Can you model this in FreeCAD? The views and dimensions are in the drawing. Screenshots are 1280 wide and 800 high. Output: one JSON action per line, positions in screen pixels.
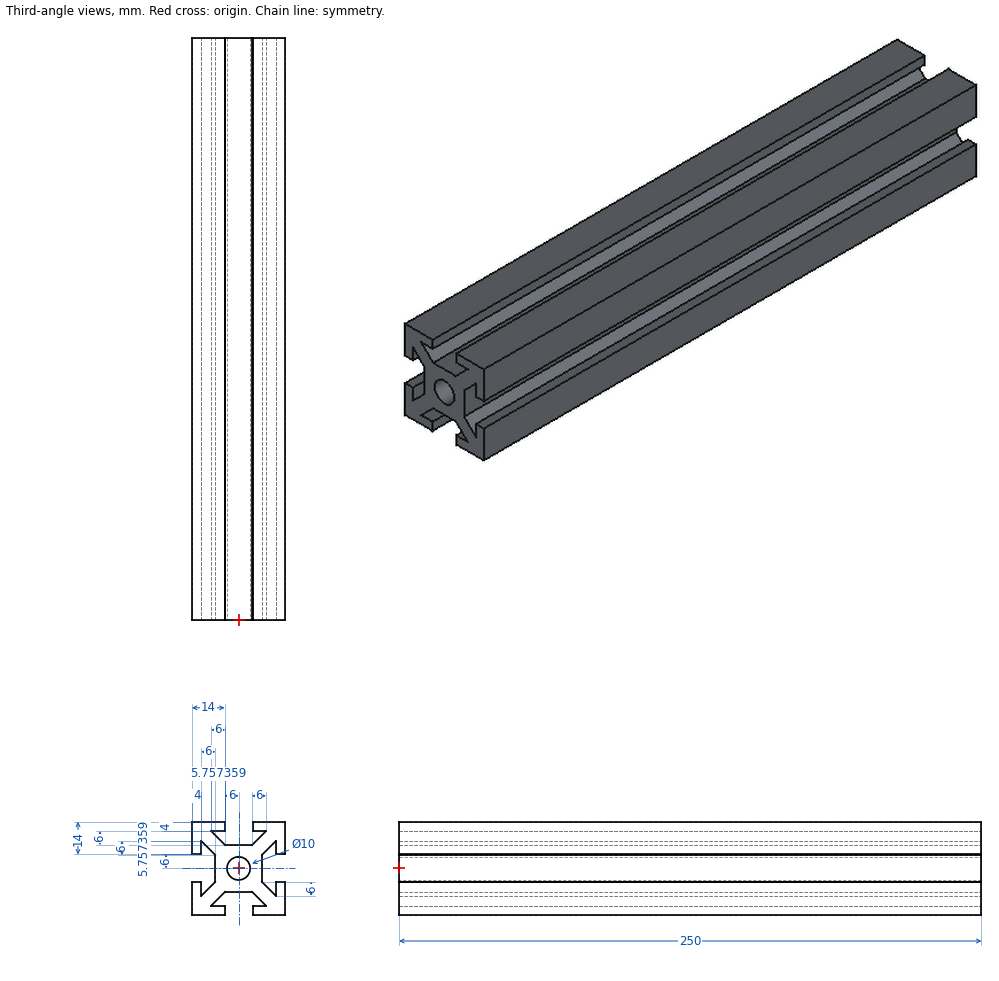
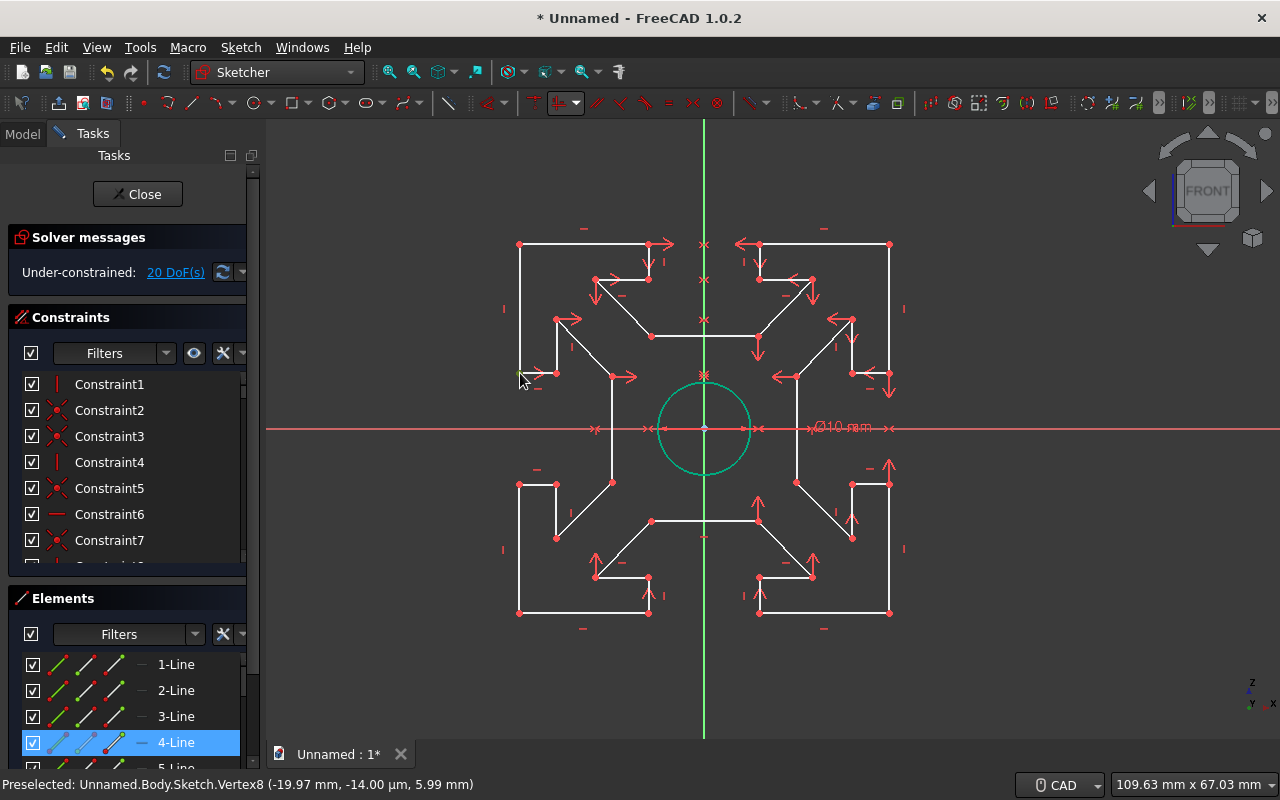
{"action": "left_click", "coordinate": [519, 485]}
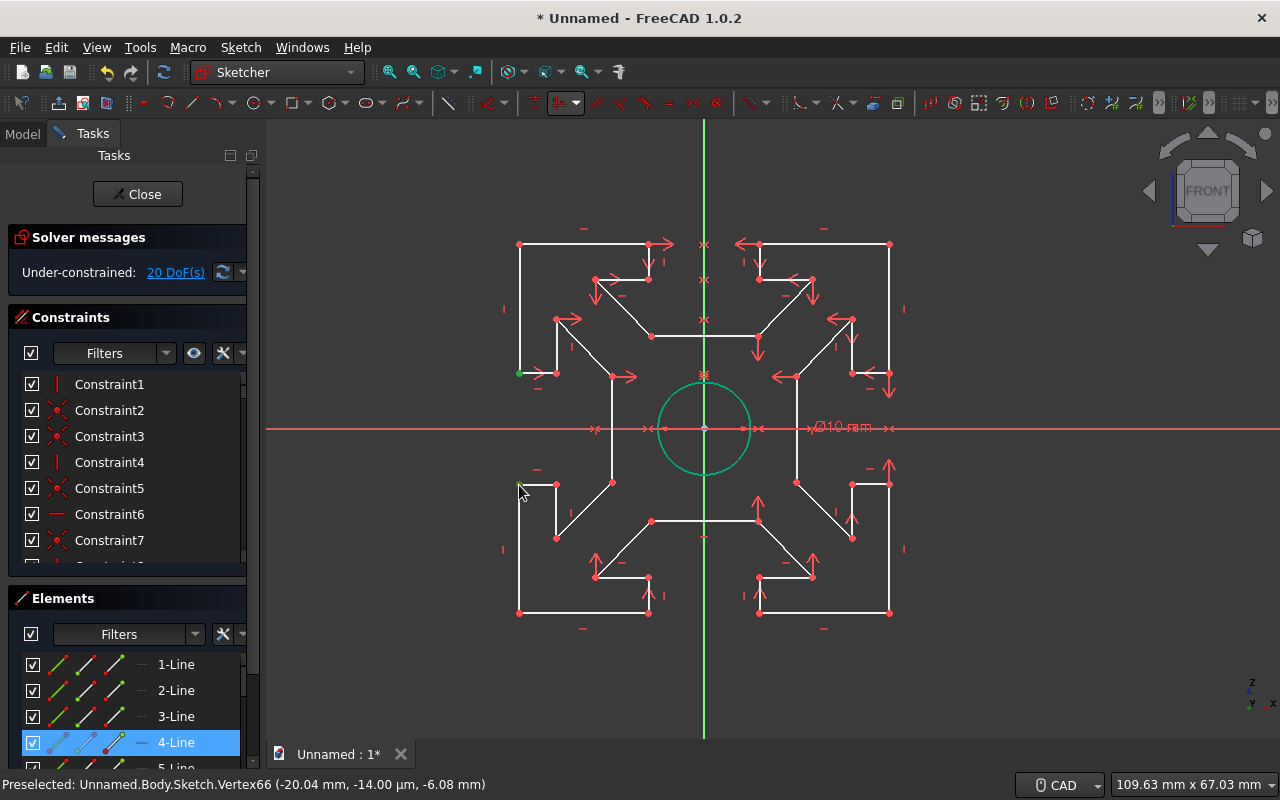
{"action": "left_click", "coordinate": [353, 429]}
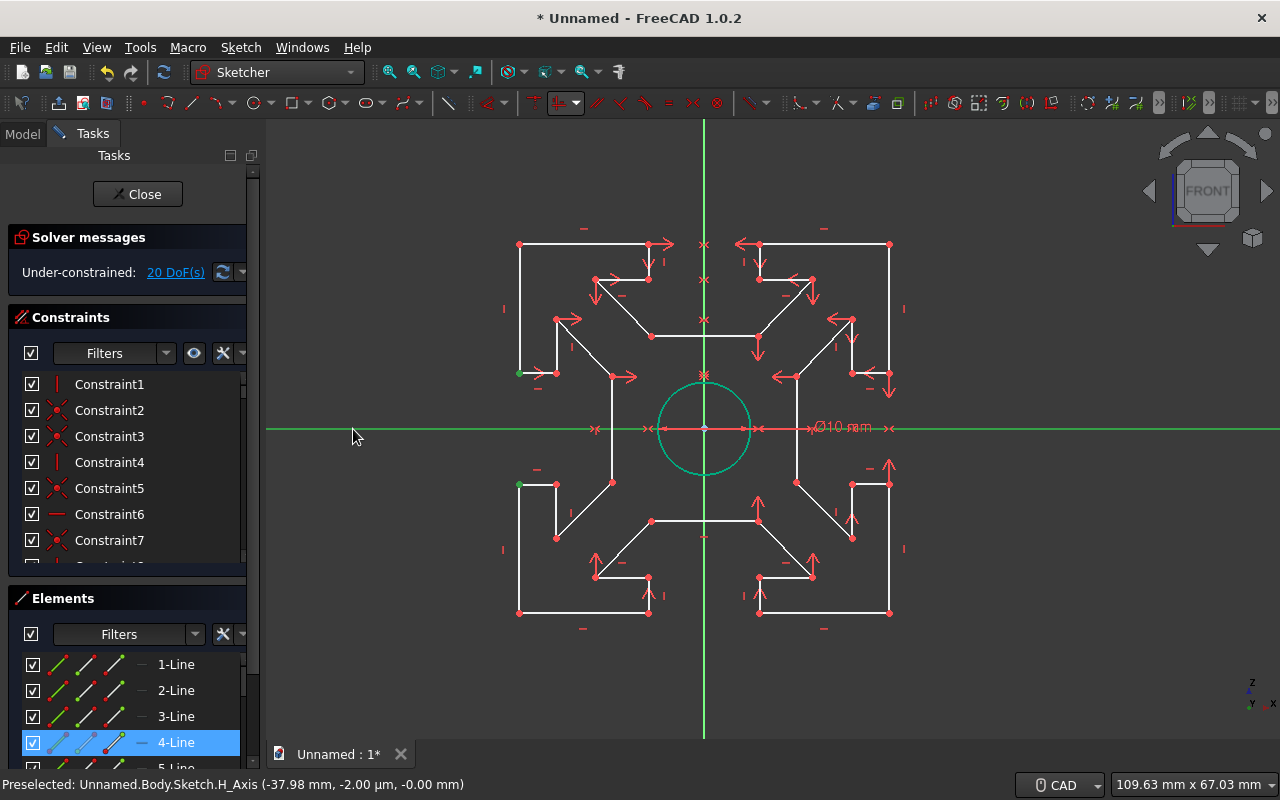
{"action": "left_click", "coordinate": [694, 104]}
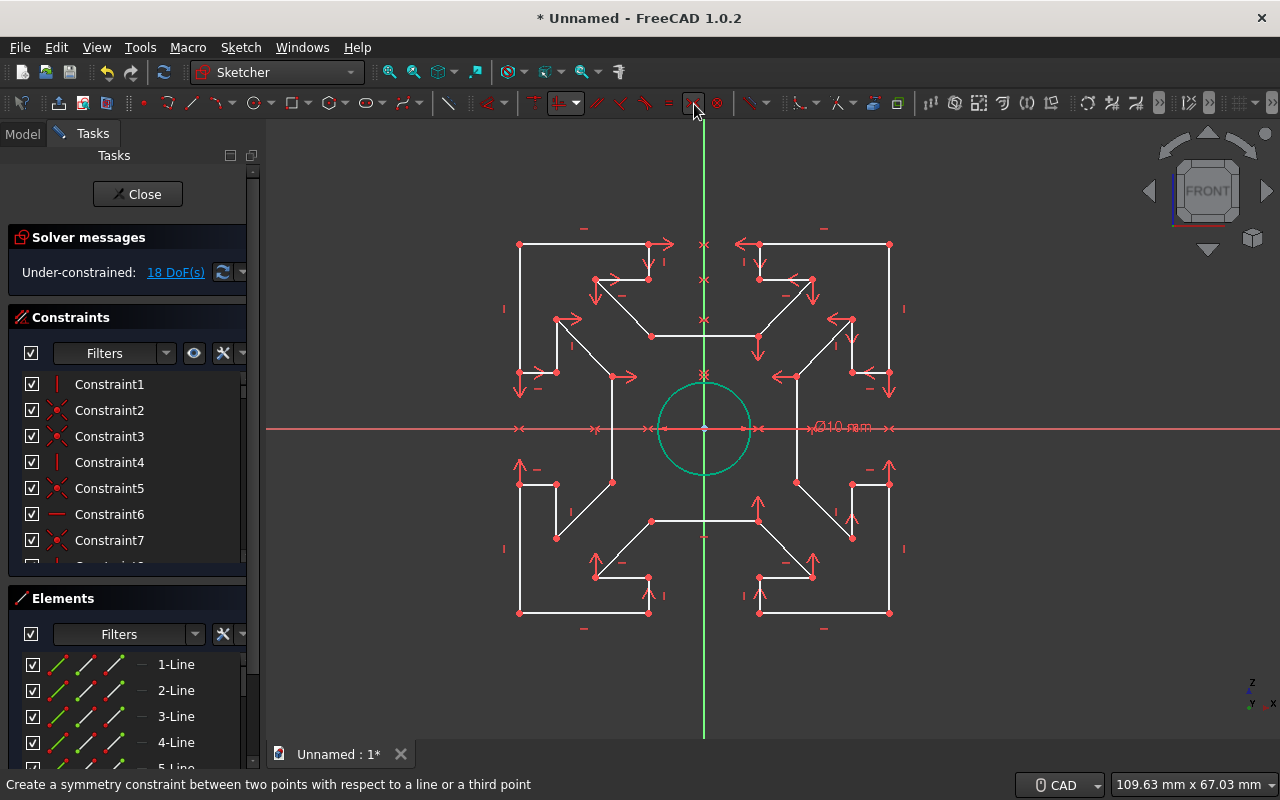
{"action": "left_click", "coordinate": [557, 319]}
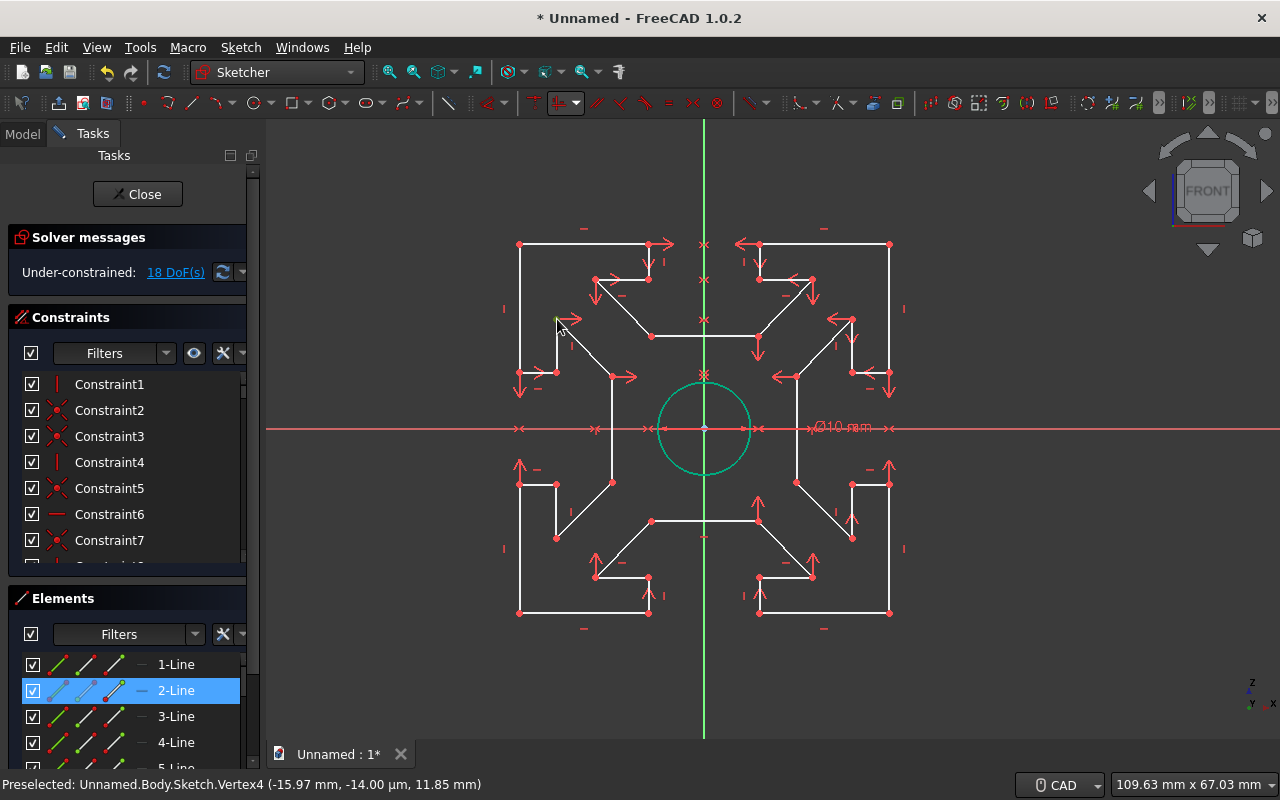
{"action": "left_click", "coordinate": [556, 539]}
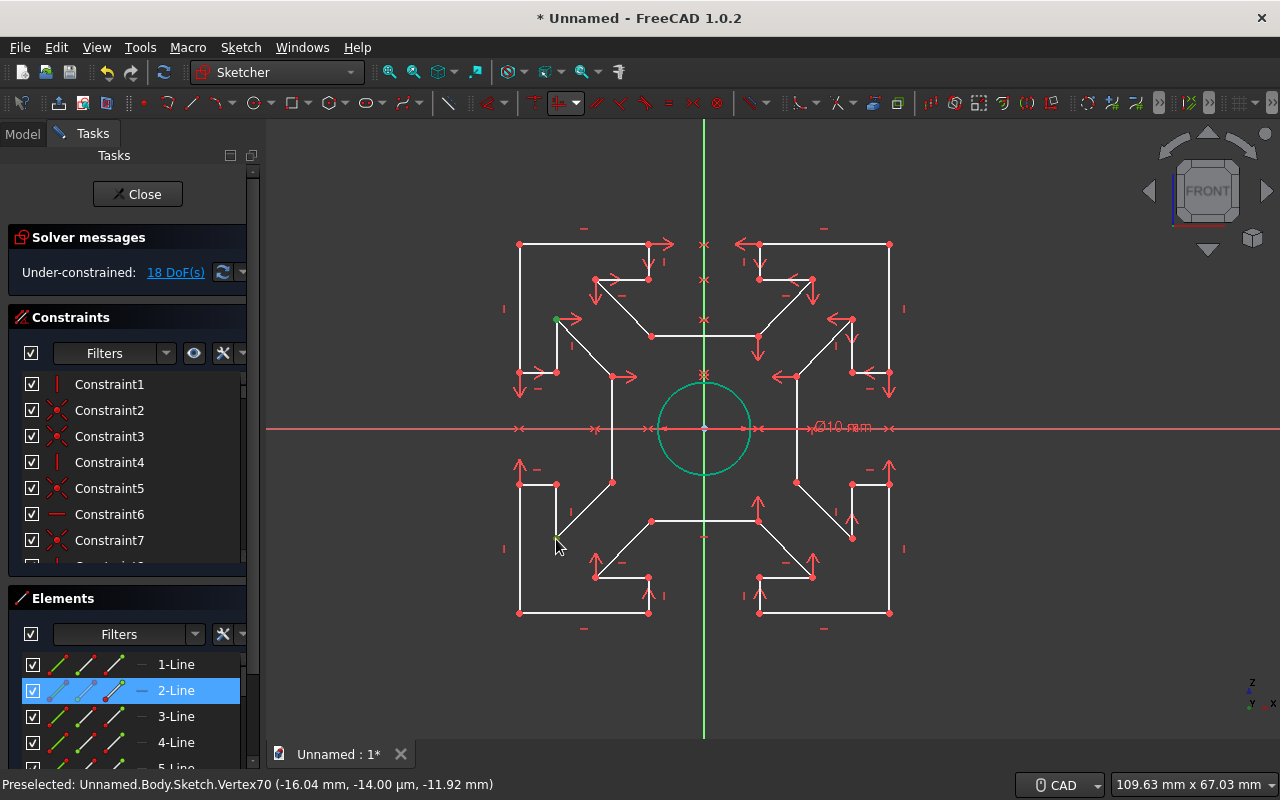
{"action": "left_click", "coordinate": [353, 429]}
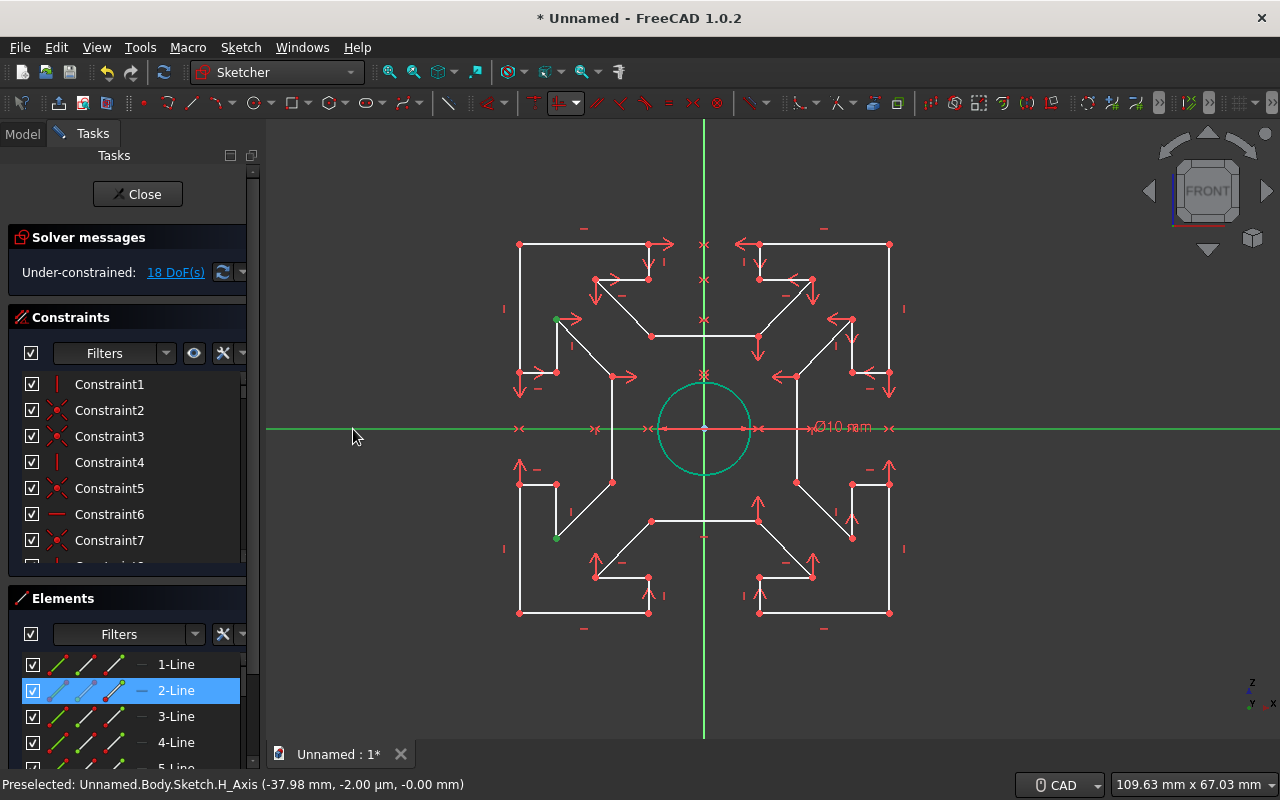
{"action": "left_click", "coordinate": [694, 104]}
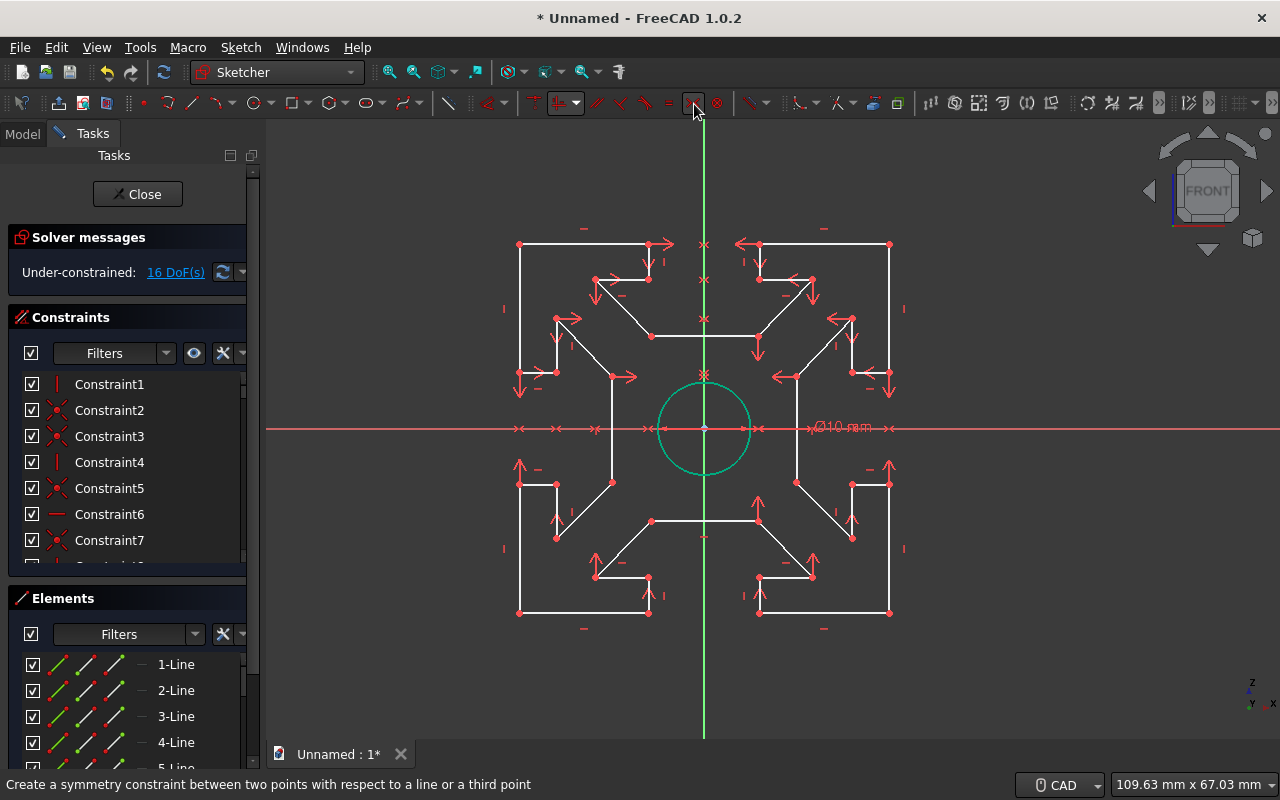
{"action": "left_click", "coordinate": [488, 104]}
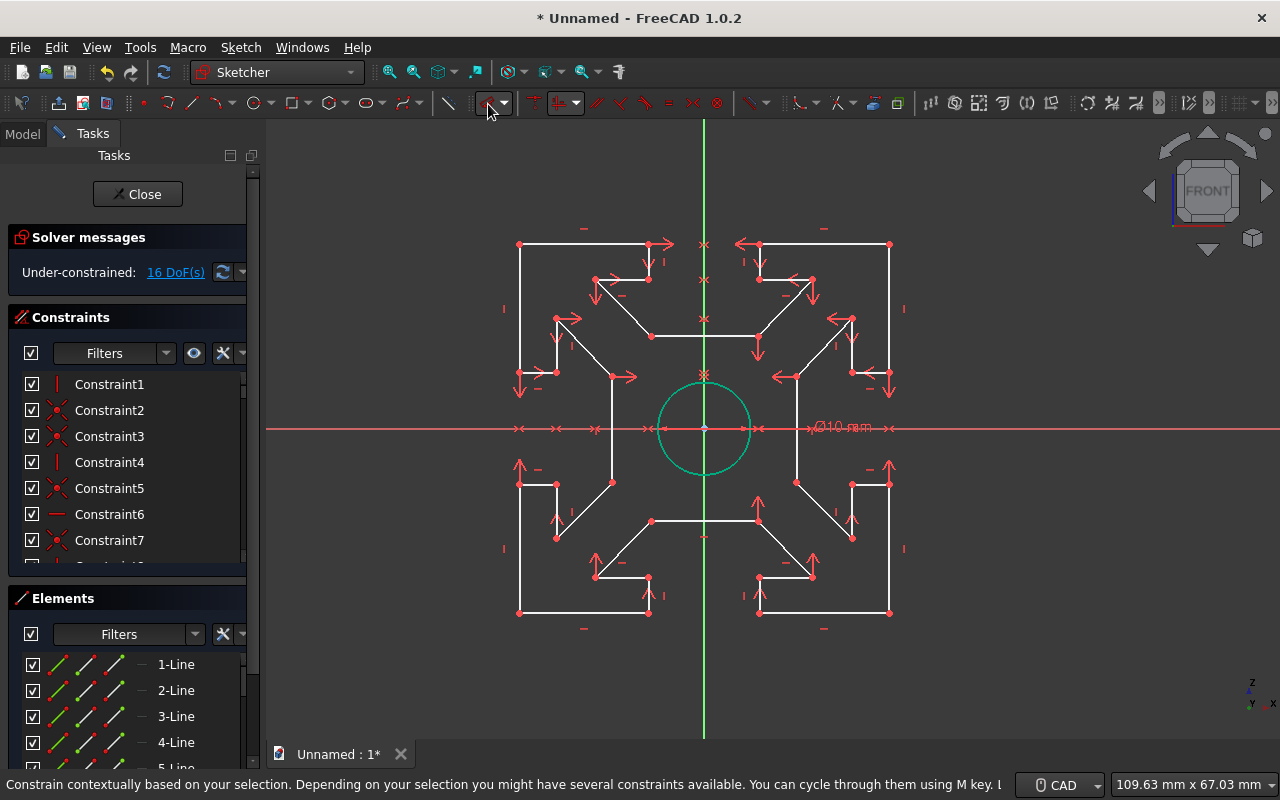
{"action": "scroll", "coordinate": [546, 373], "scroll_direction": "up", "scroll_amount": 2}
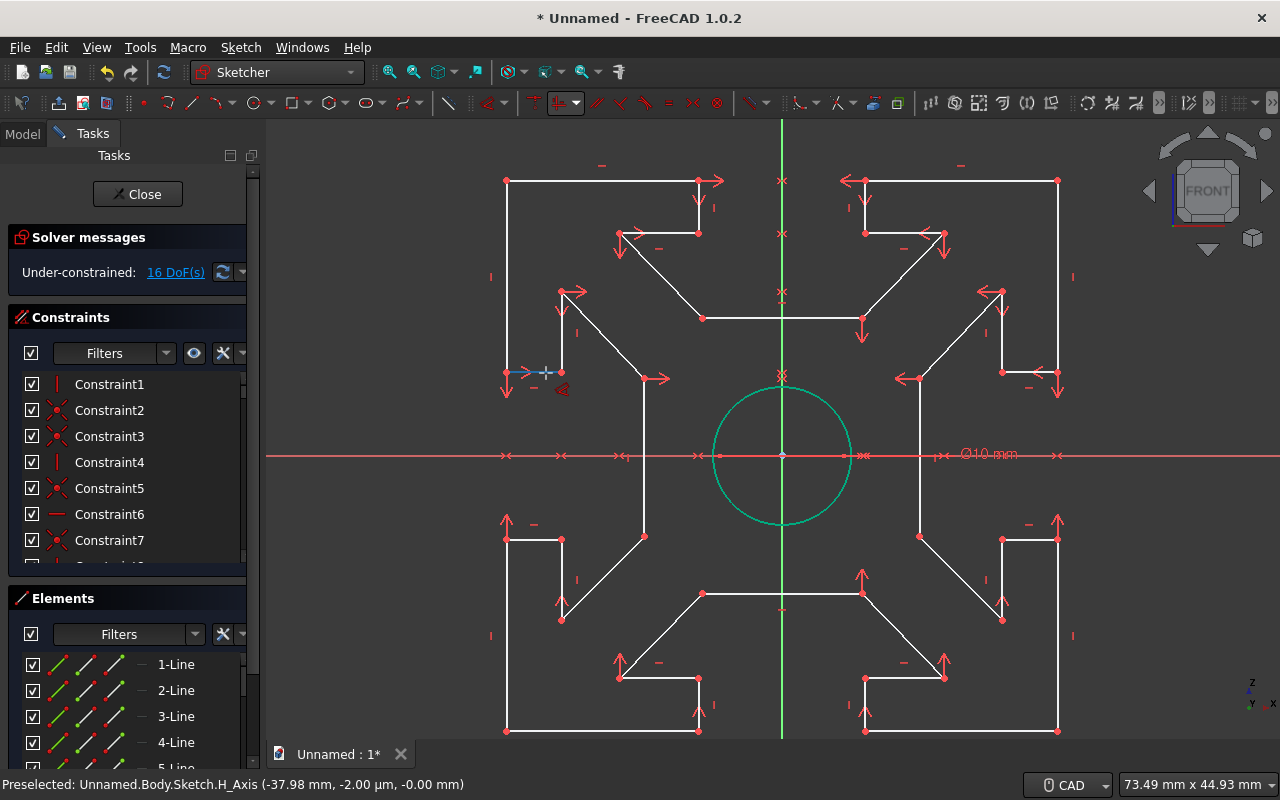
{"action": "left_click", "coordinate": [545, 372]}
{"action": "left_click", "coordinate": [534, 338]}